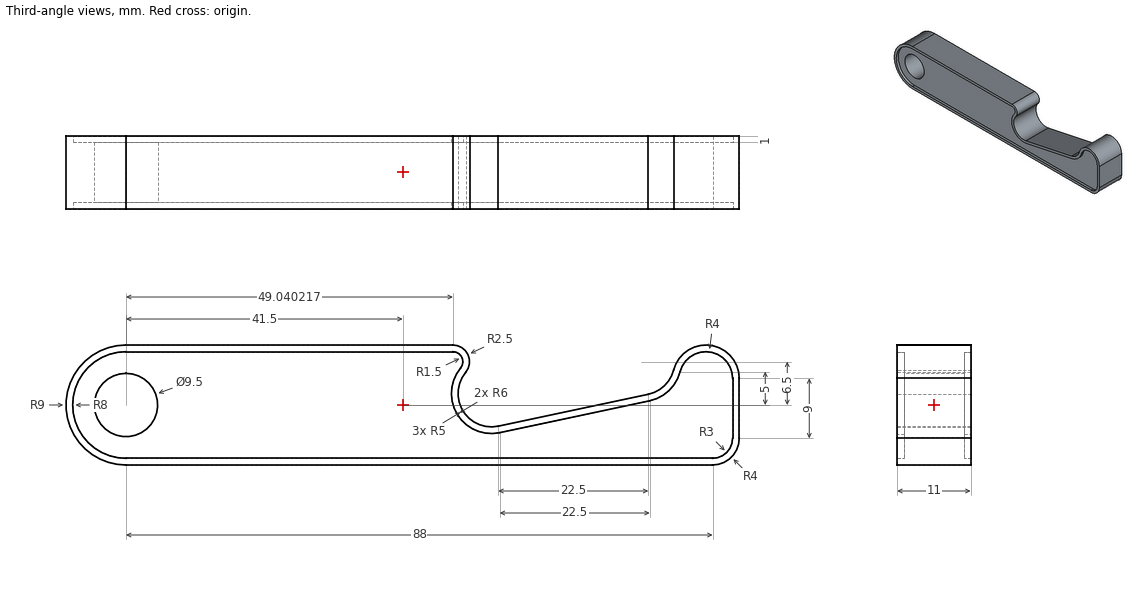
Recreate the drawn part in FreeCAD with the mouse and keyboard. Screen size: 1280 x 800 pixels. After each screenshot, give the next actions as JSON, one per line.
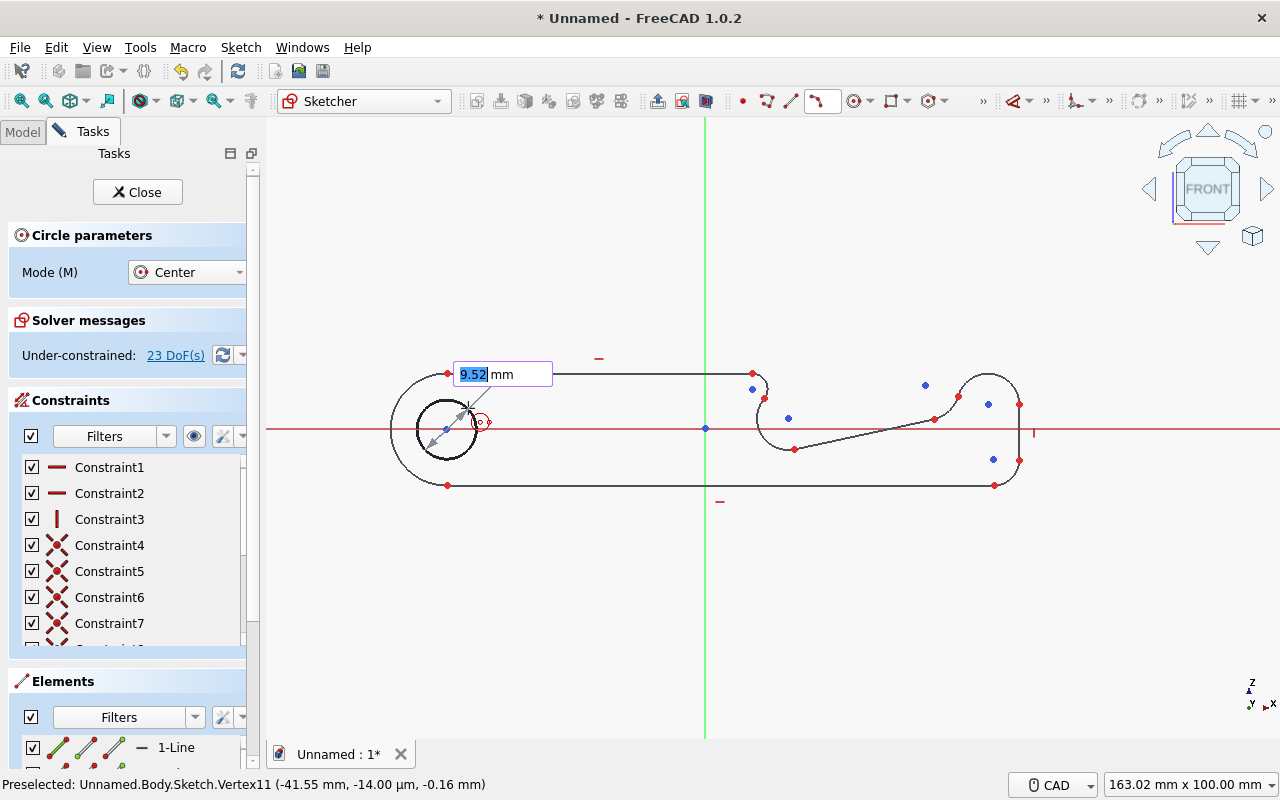
{"action": "type", "text": "9.5"}
{"action": "key", "text": "Return"}
{"action": "key", "text": "Escape"}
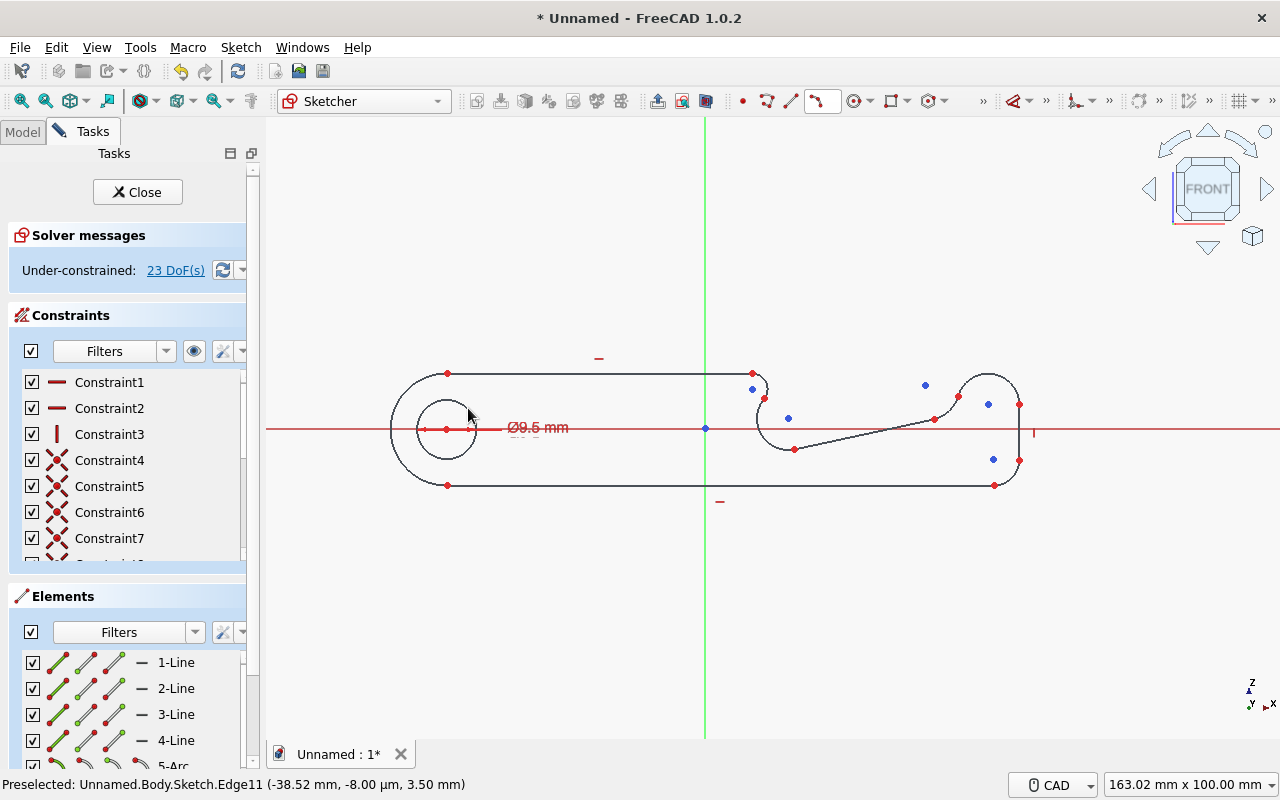
{"action": "left_click", "coordinate": [830, 486]}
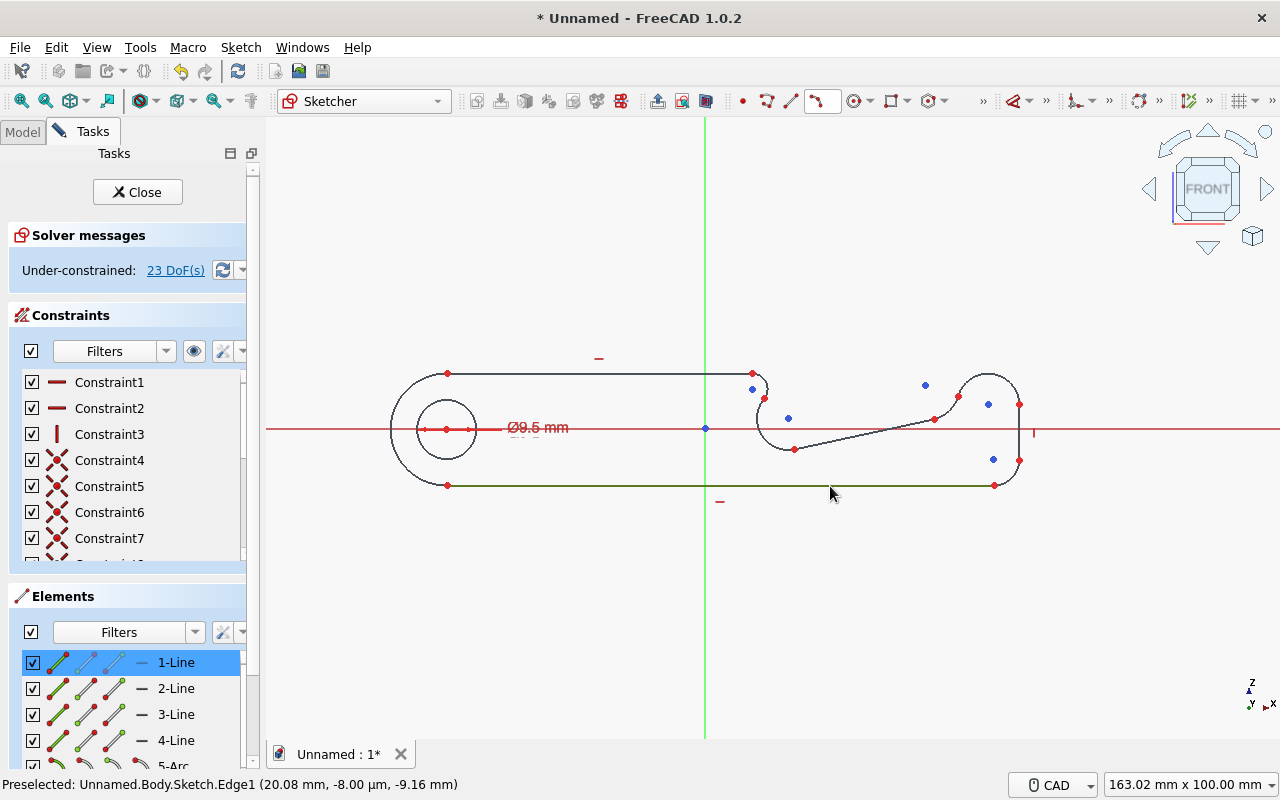
{"action": "left_click", "coordinate": [401, 396]}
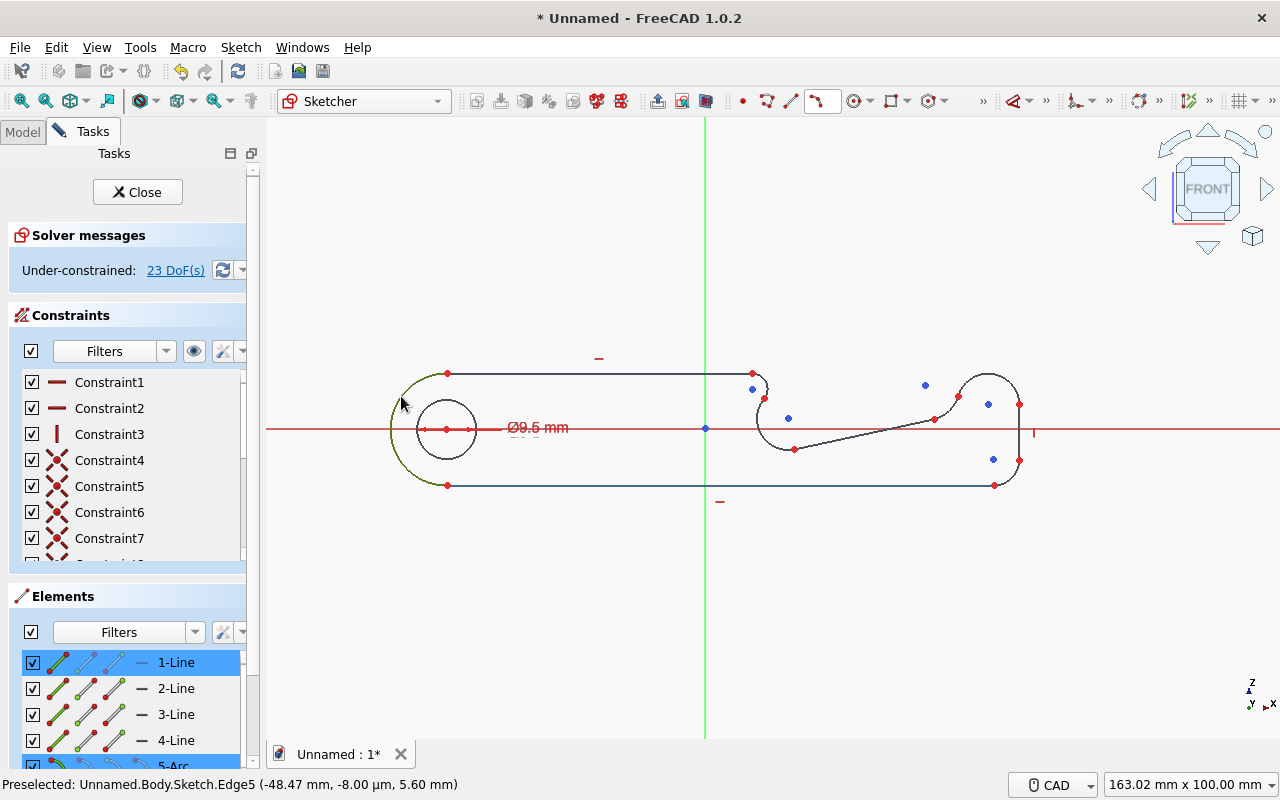
{"action": "key", "text": "t"}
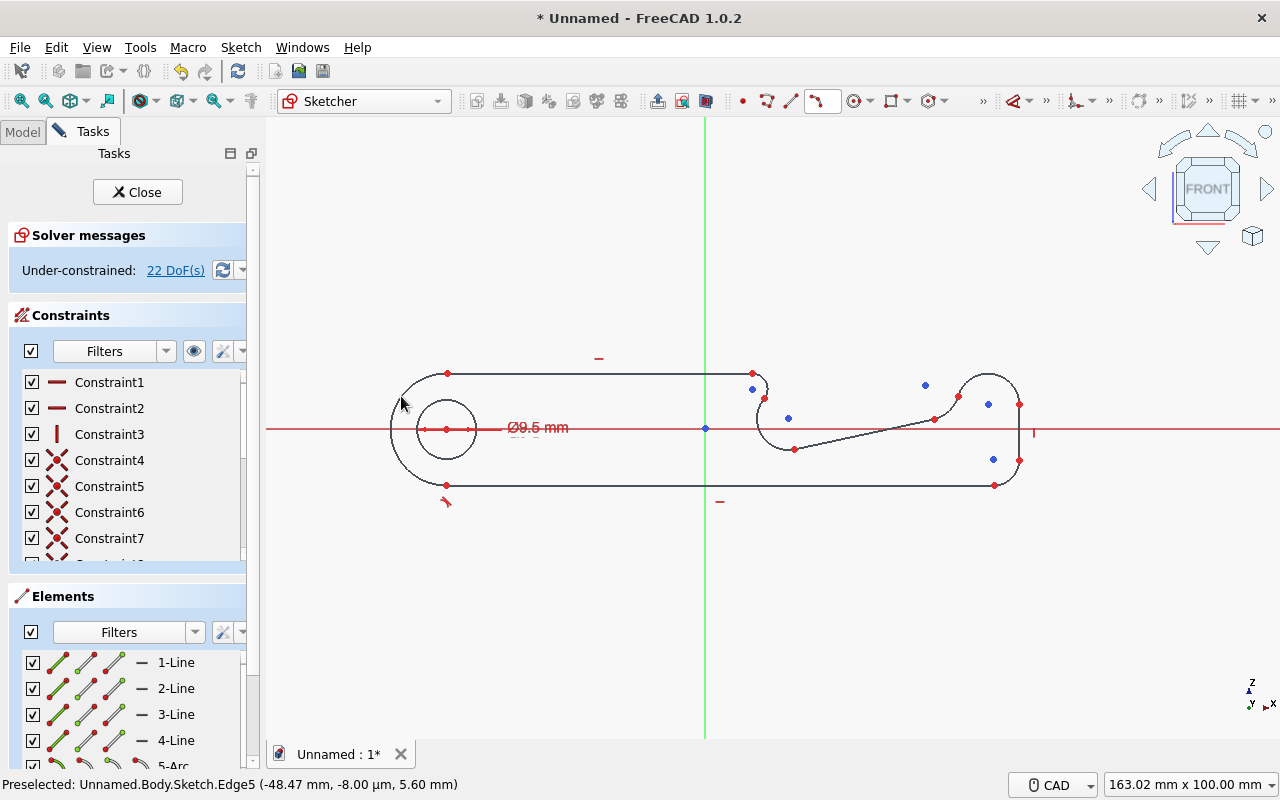
{"action": "left_click", "coordinate": [830, 486]}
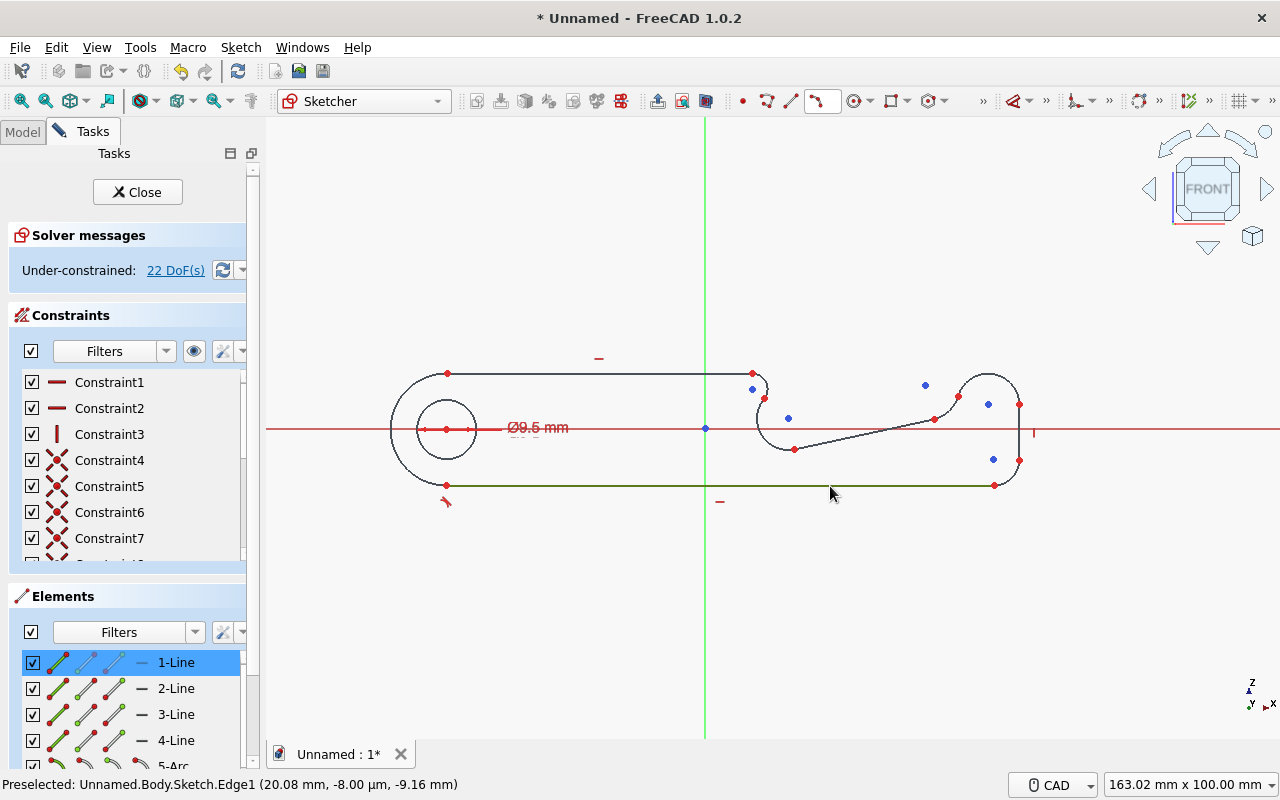
{"action": "left_click", "coordinate": [1005, 483]}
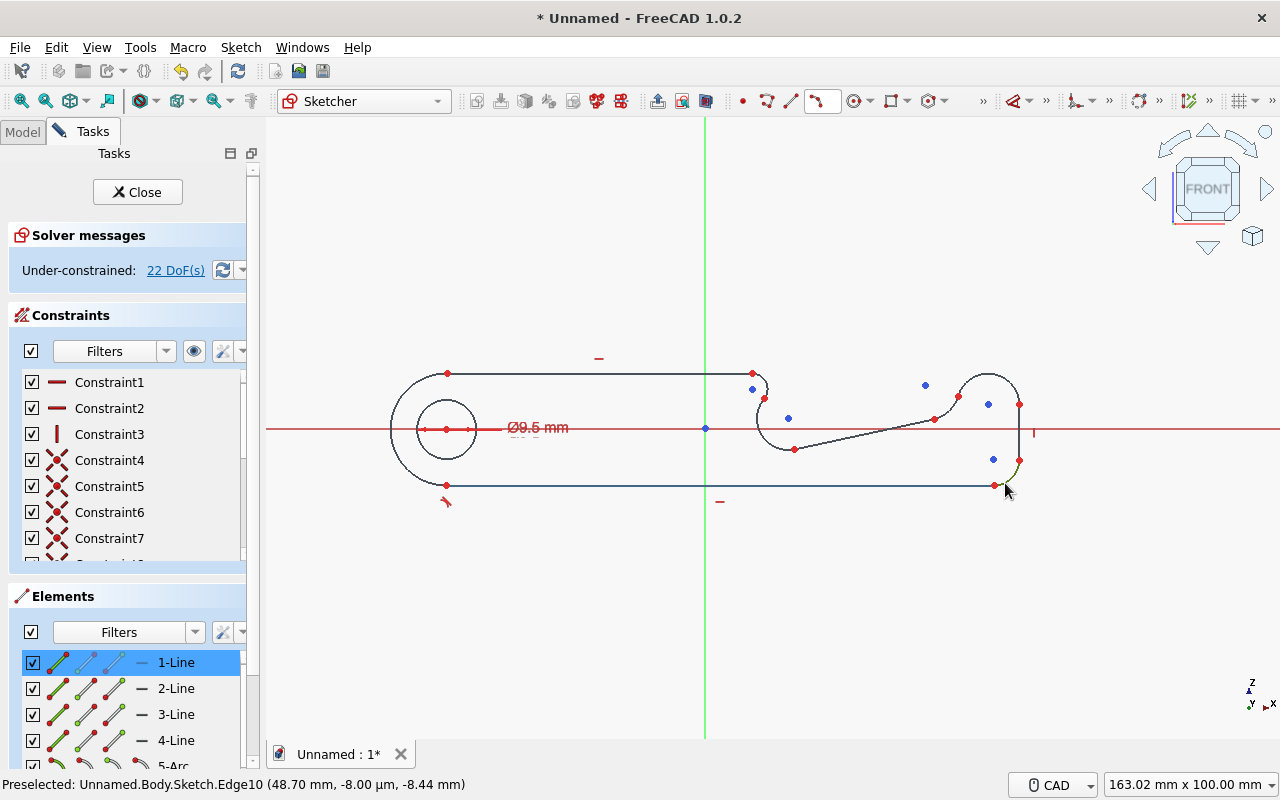
{"action": "key", "text": "t"}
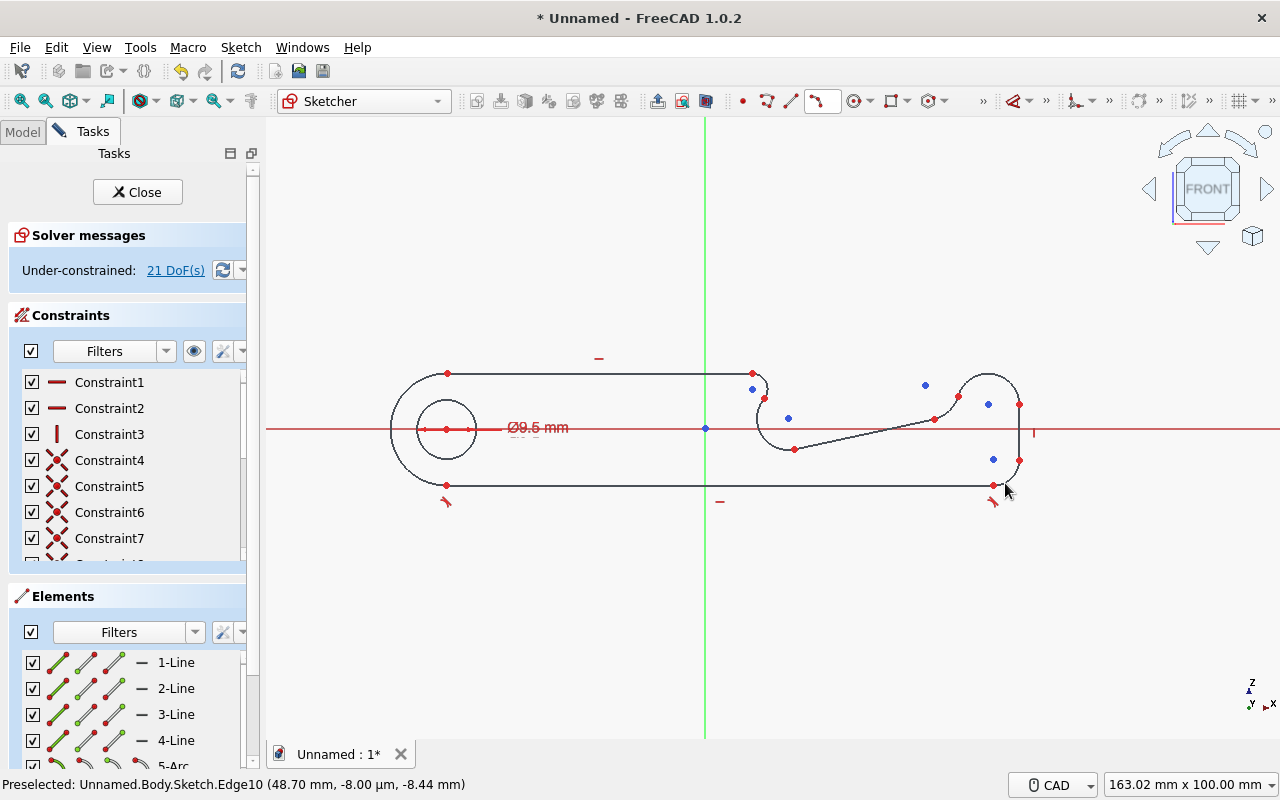
{"action": "left_click", "coordinate": [539, 374]}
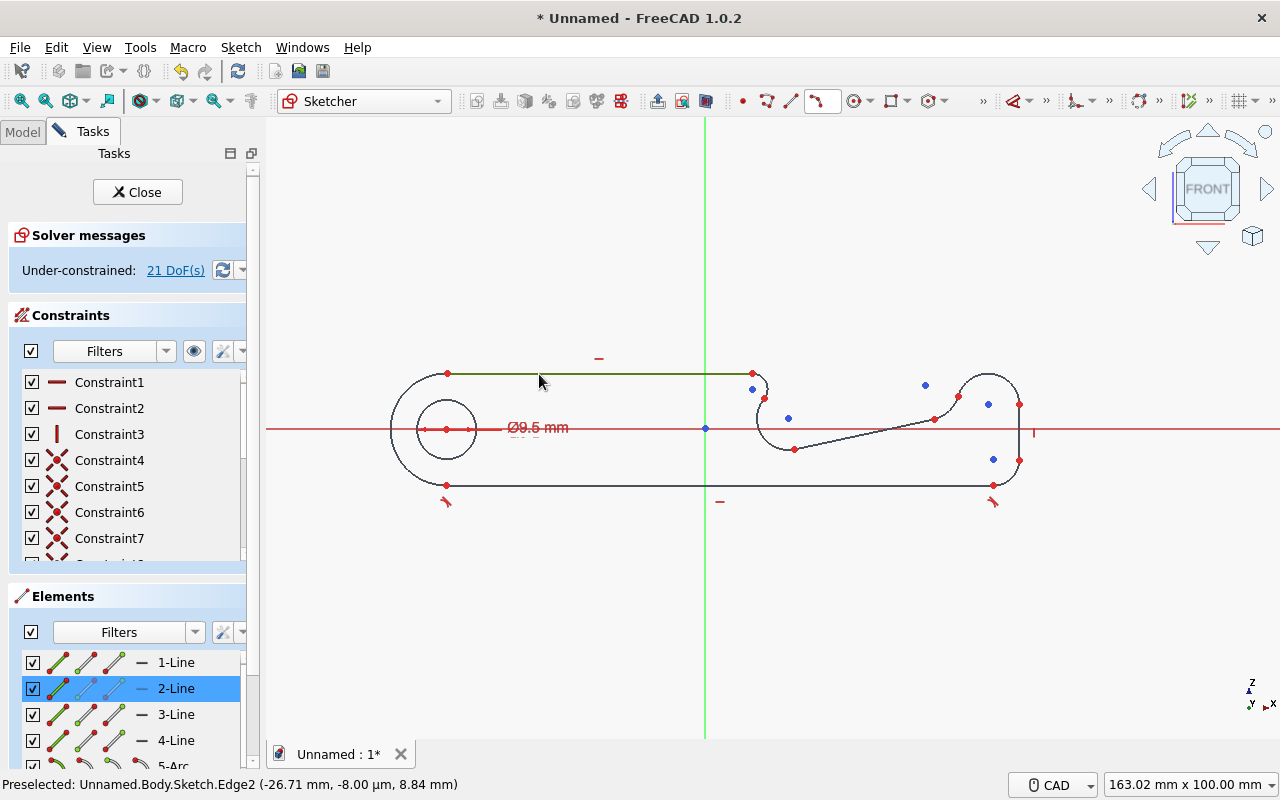
{"action": "left_click", "coordinate": [402, 396]}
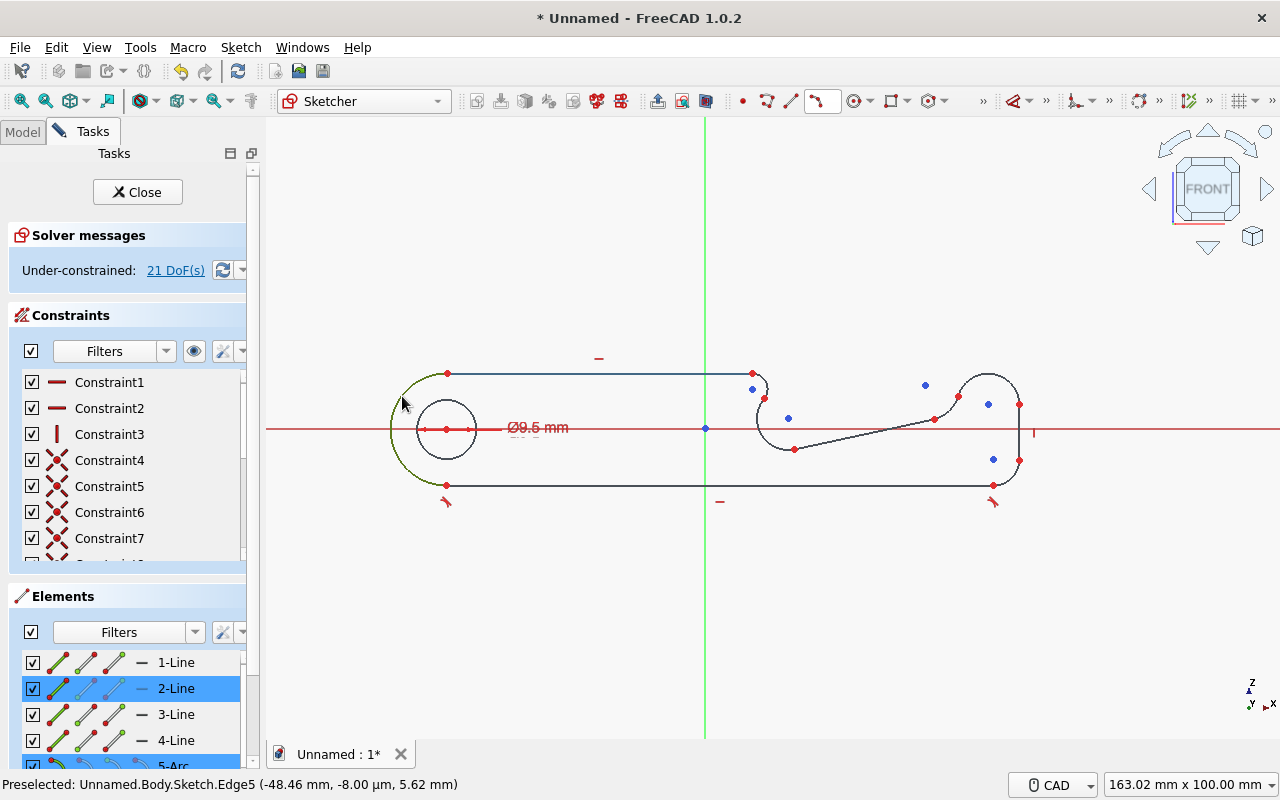
{"action": "key", "text": "t"}